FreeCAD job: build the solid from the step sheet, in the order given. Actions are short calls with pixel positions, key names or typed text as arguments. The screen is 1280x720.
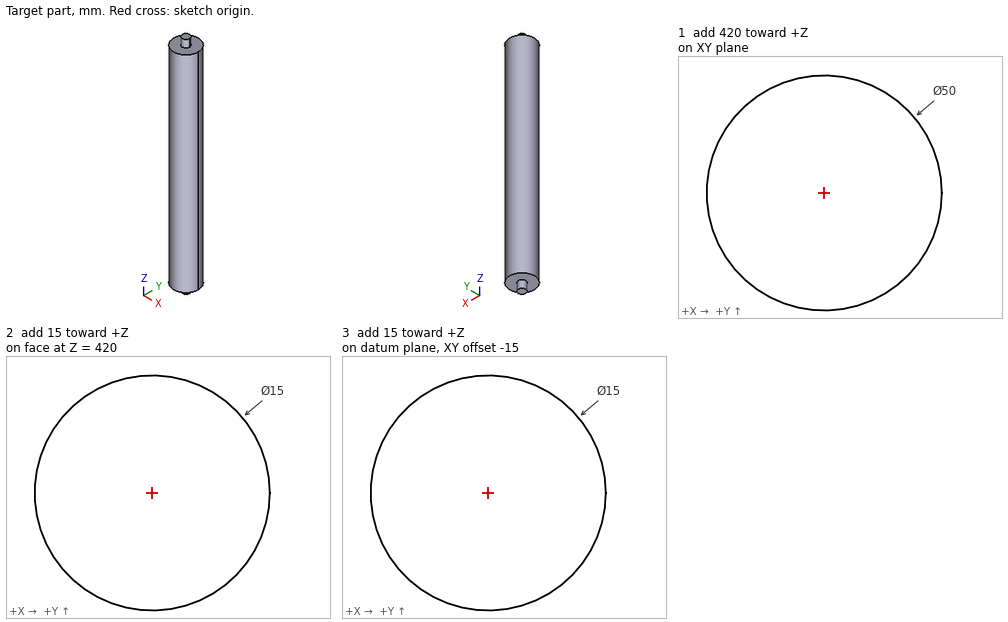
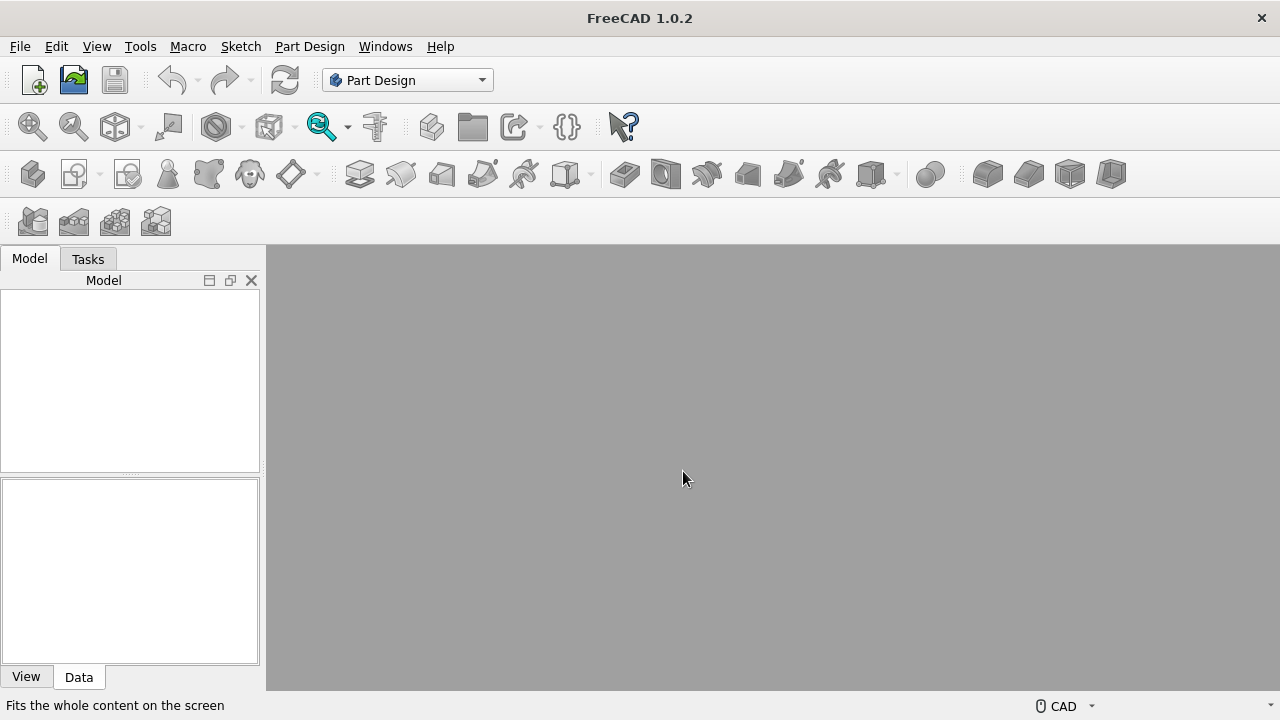
key(ctrl+n)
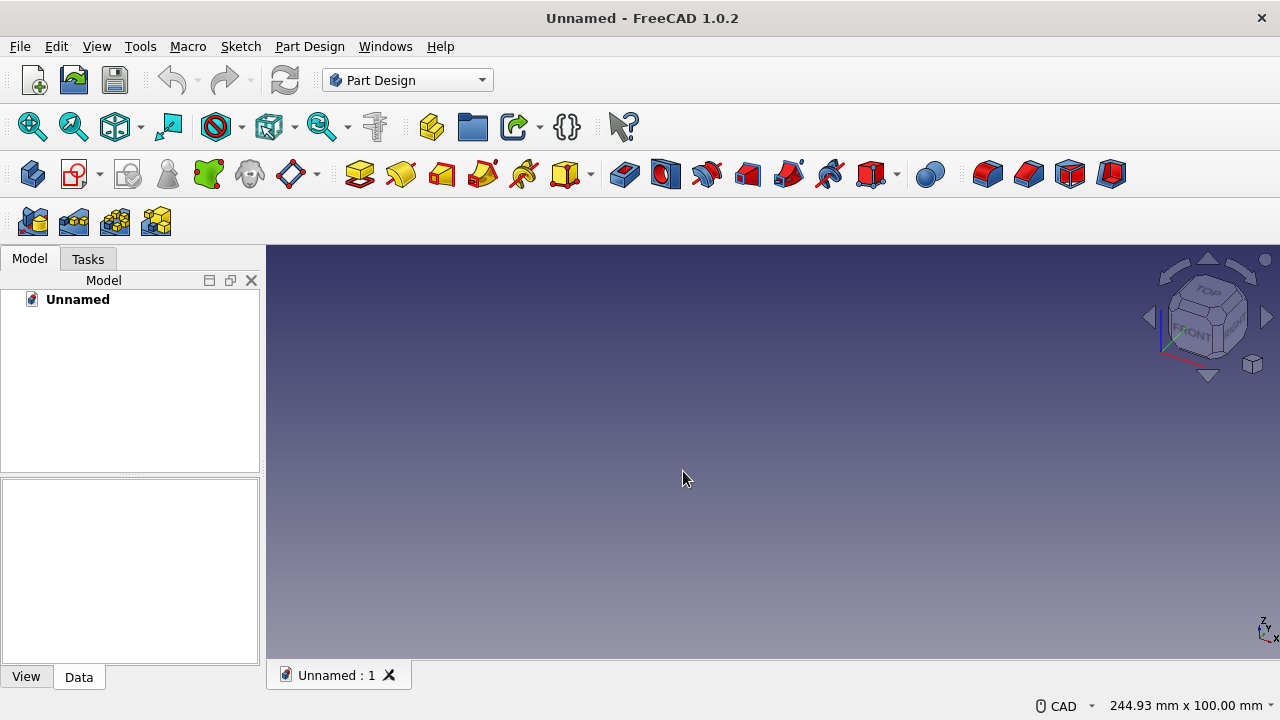
click(74, 174)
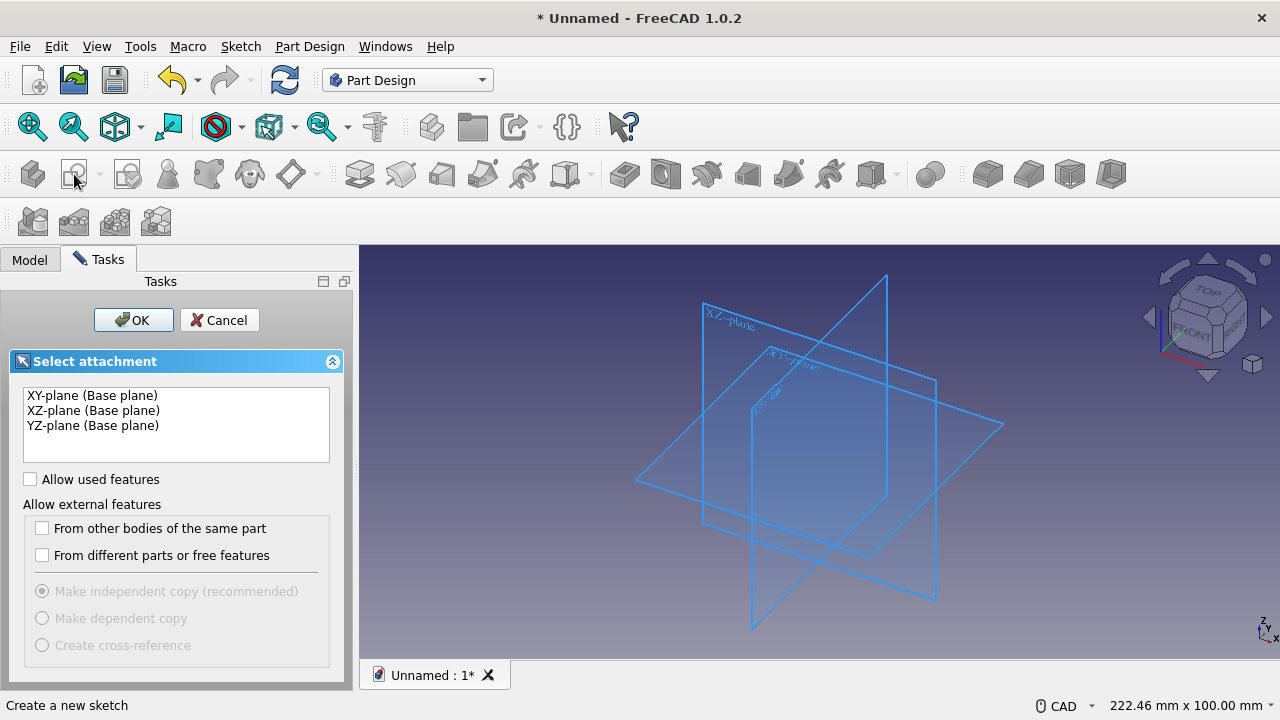
click(84, 396)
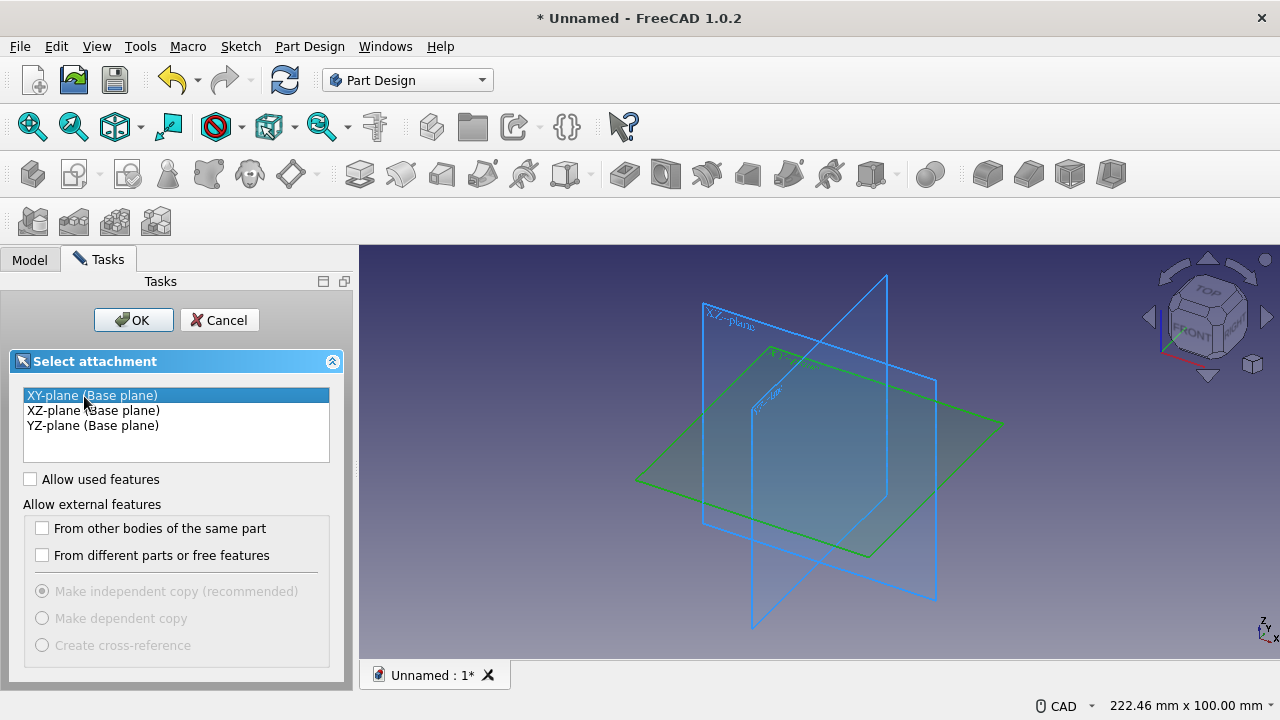
click(134, 320)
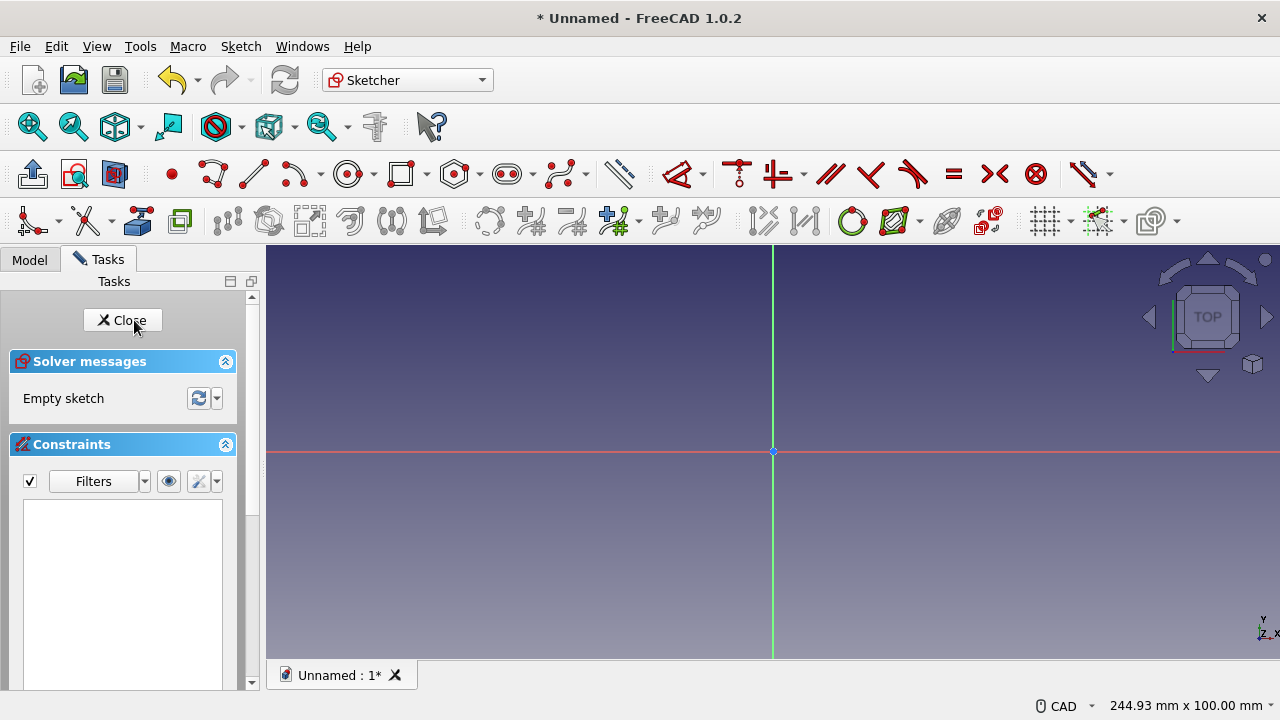
key(g)
key(c)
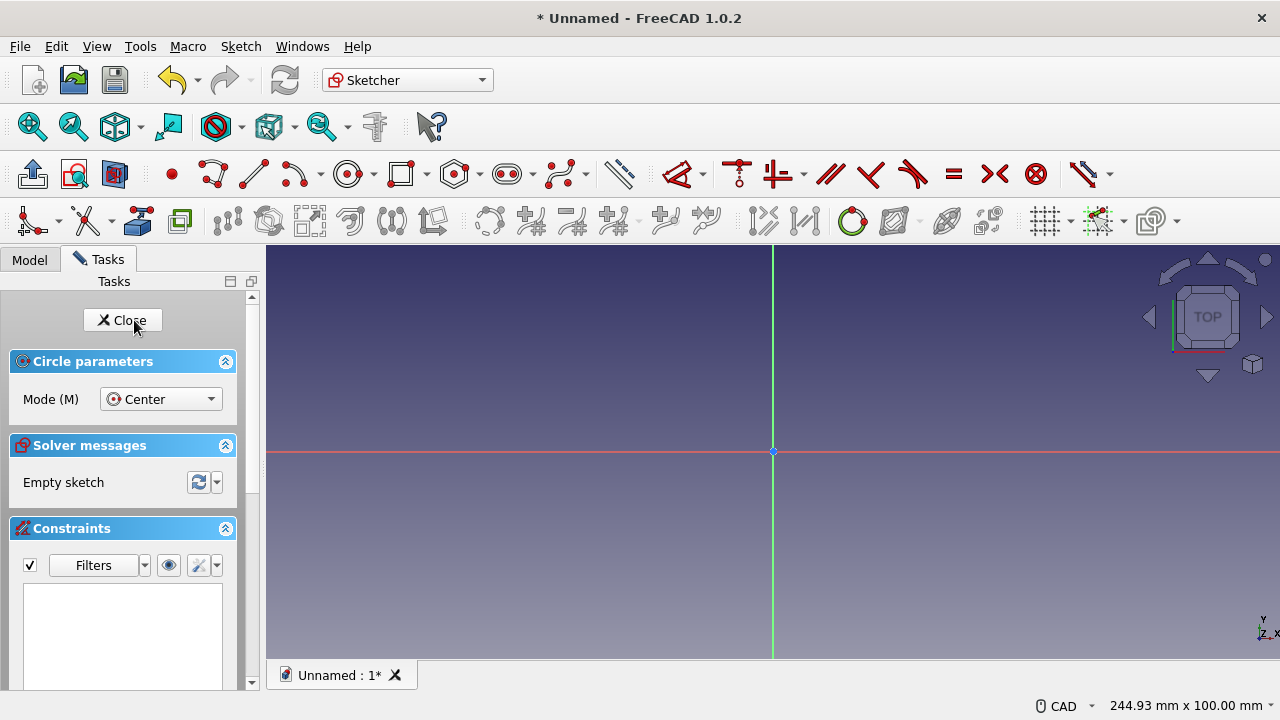
click(773, 452)
move(846, 379)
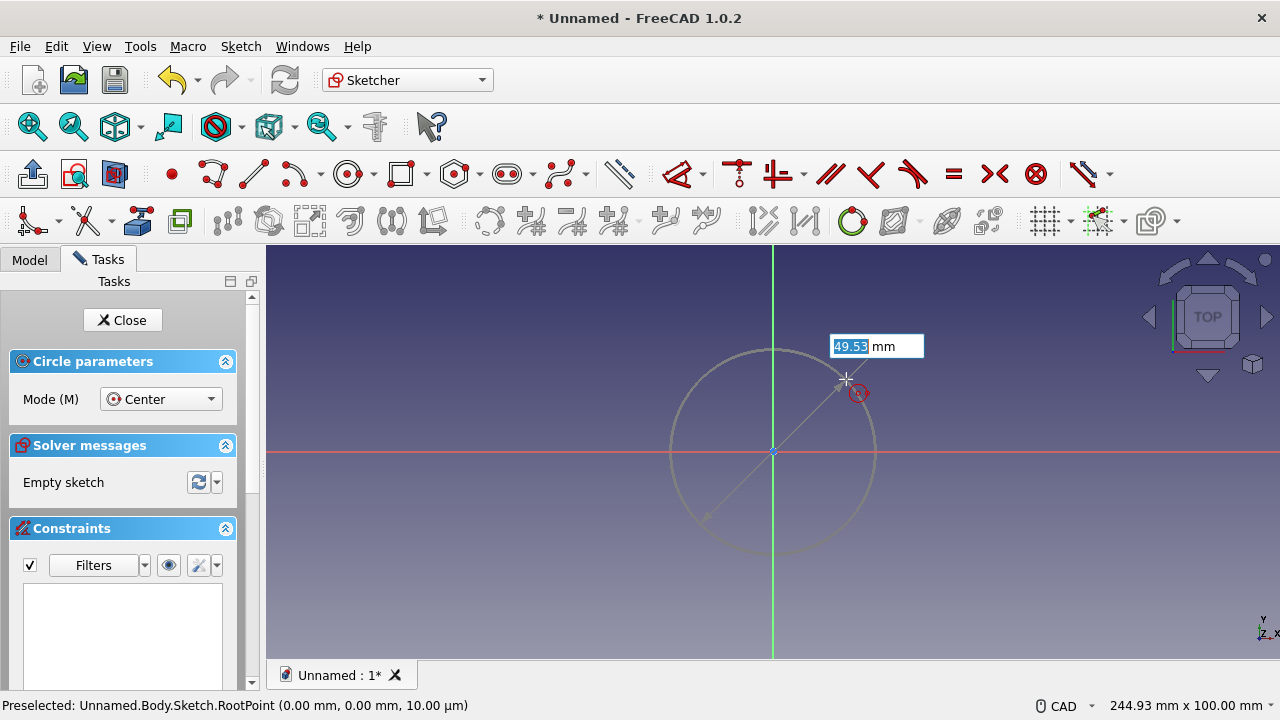
text(50)
key(Return)
key(Escape)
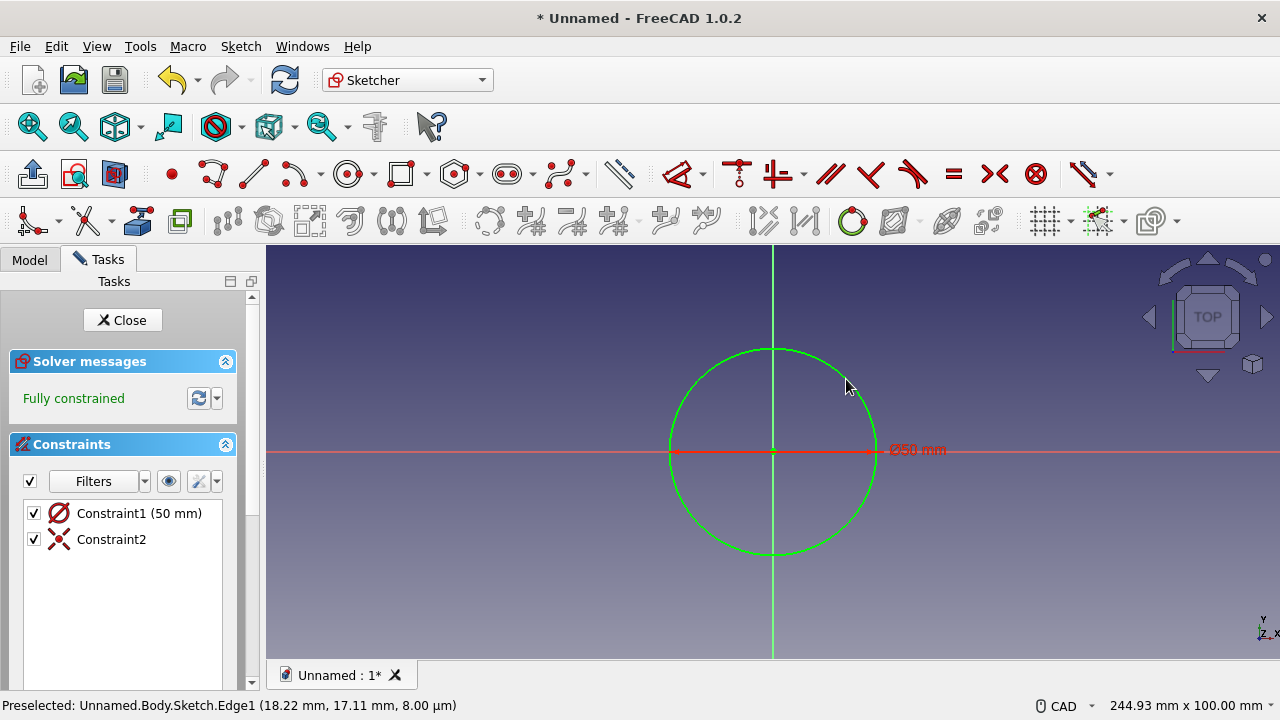
click(123, 320)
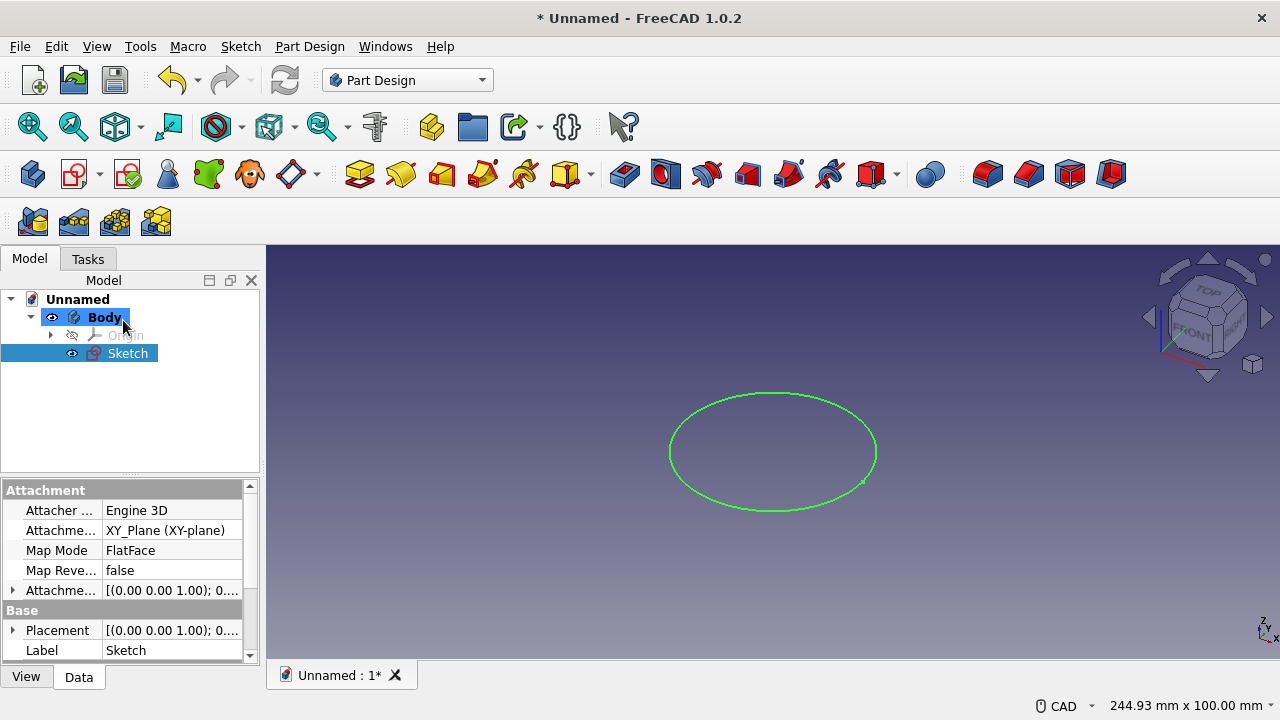
click(360, 174)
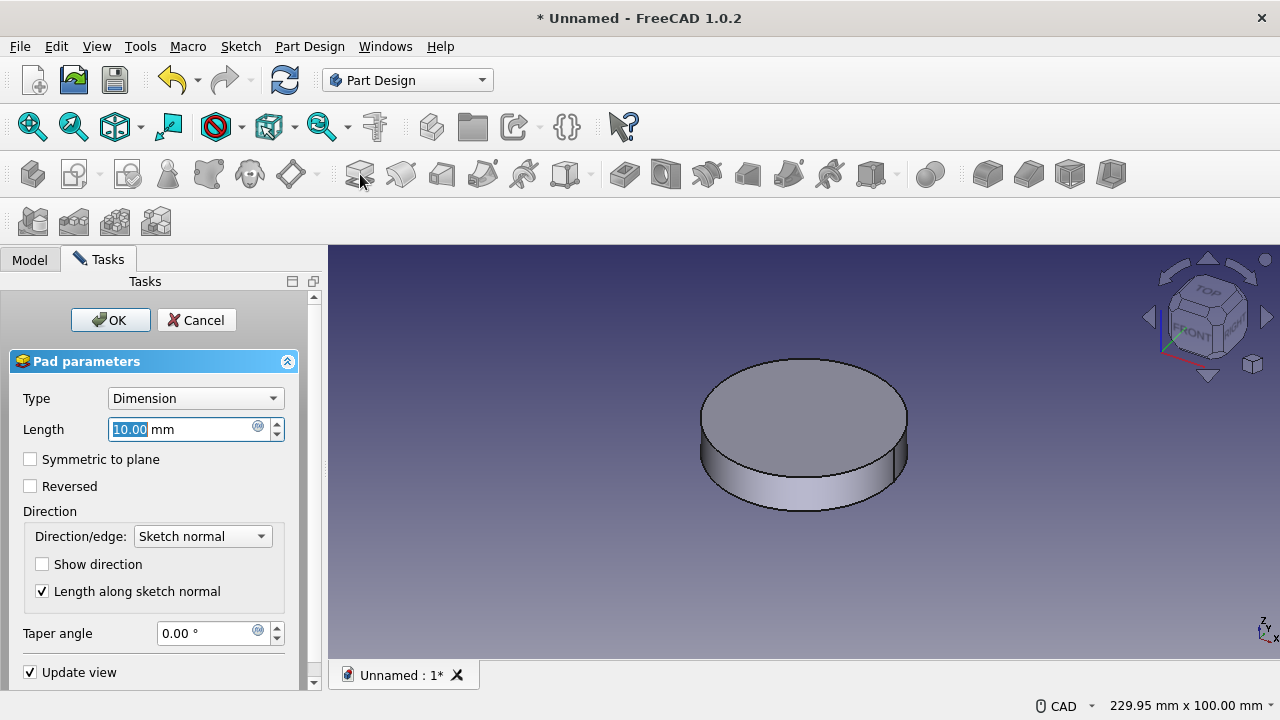
text(420)
key(Tab)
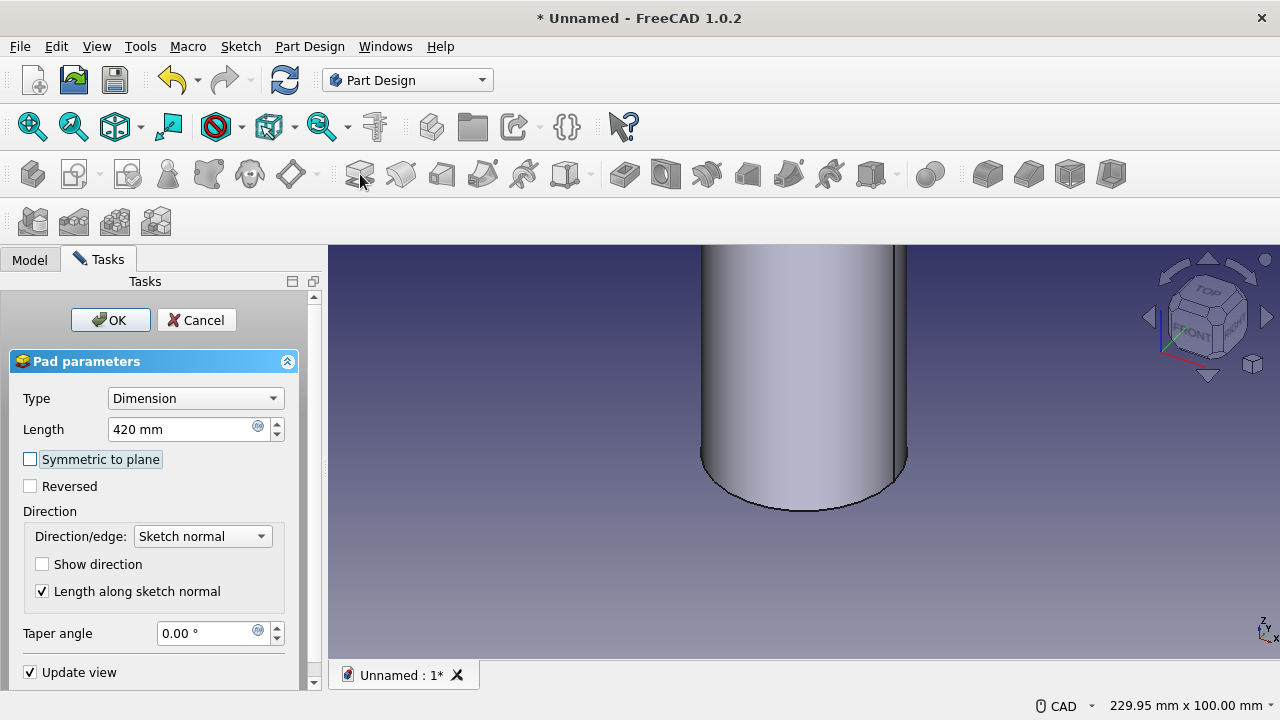
click(111, 320)